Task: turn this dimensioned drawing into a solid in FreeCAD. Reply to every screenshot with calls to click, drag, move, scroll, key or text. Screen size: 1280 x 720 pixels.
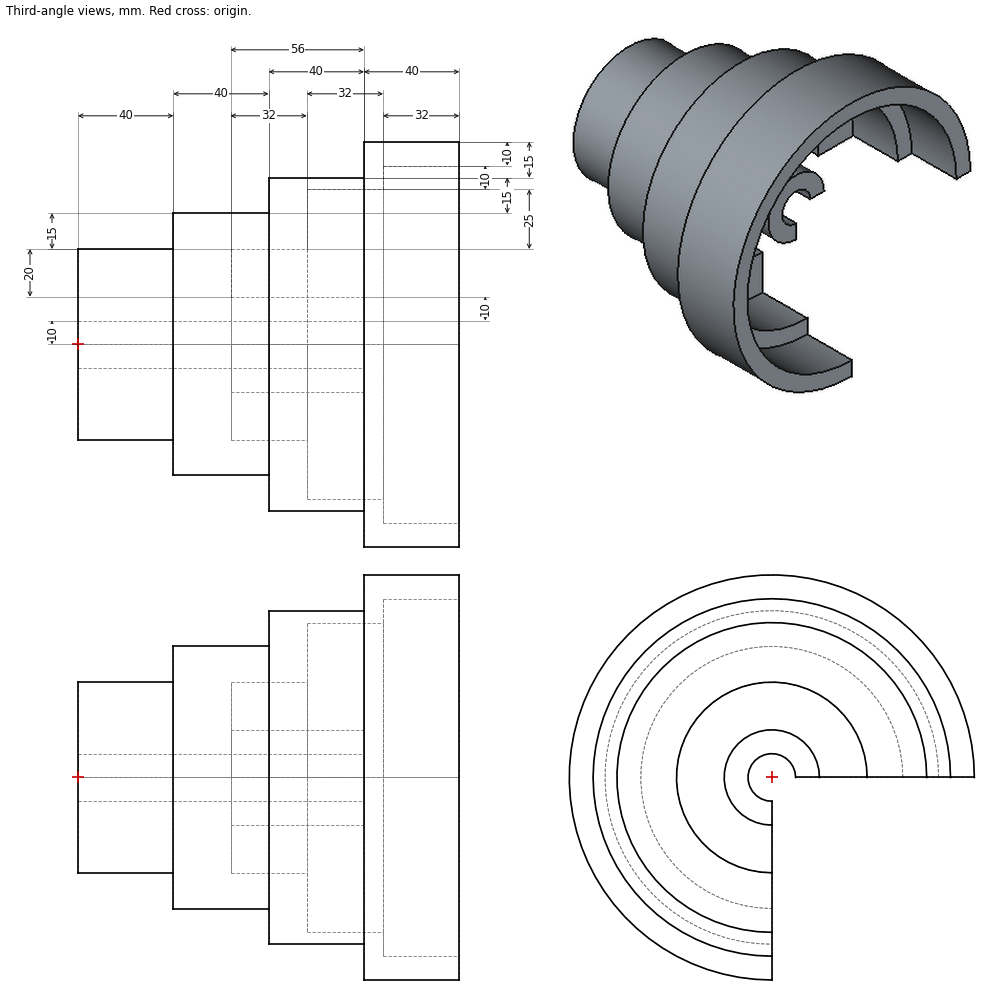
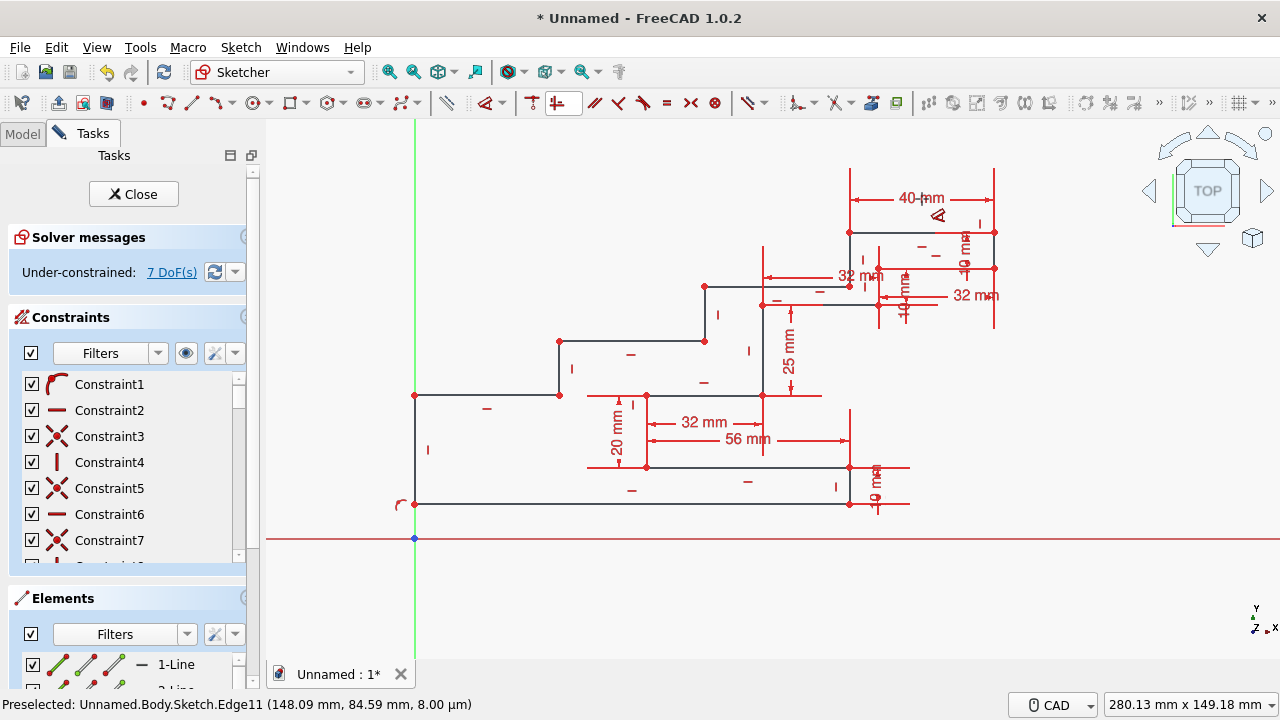
click(850, 249)
click(884, 247)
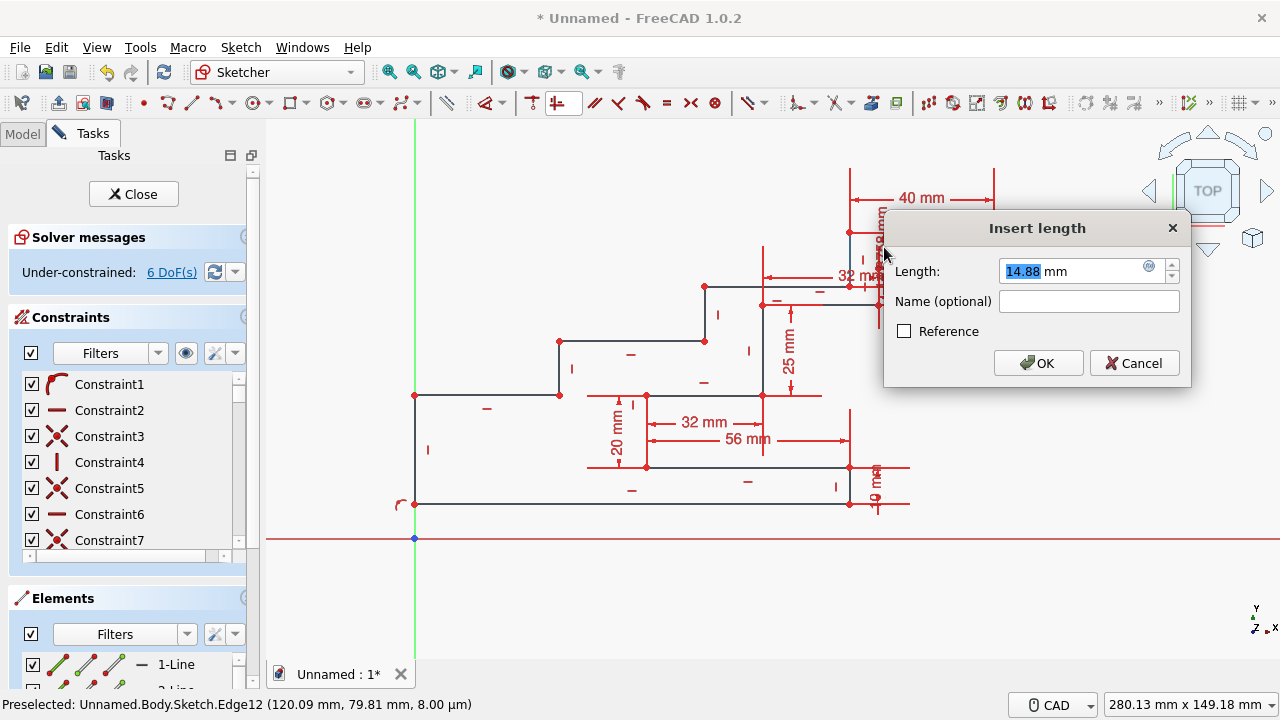
text(15)
key(Return)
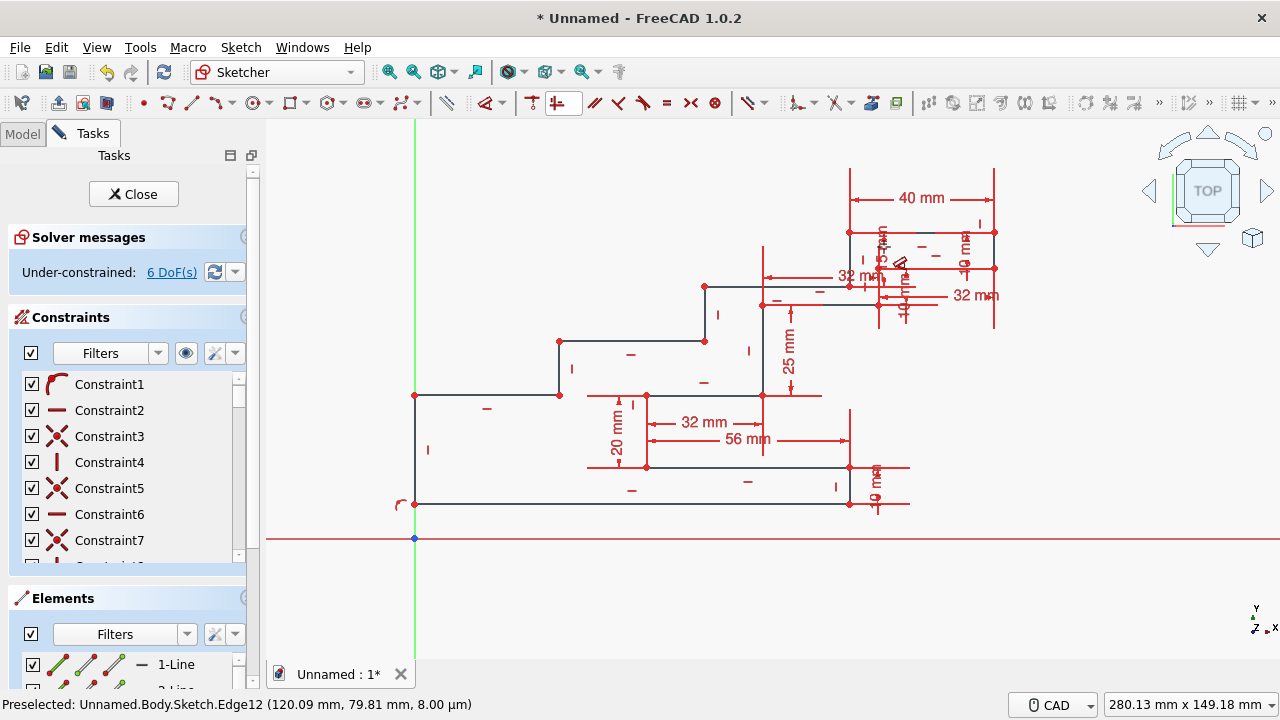
click(806, 287)
click(777, 253)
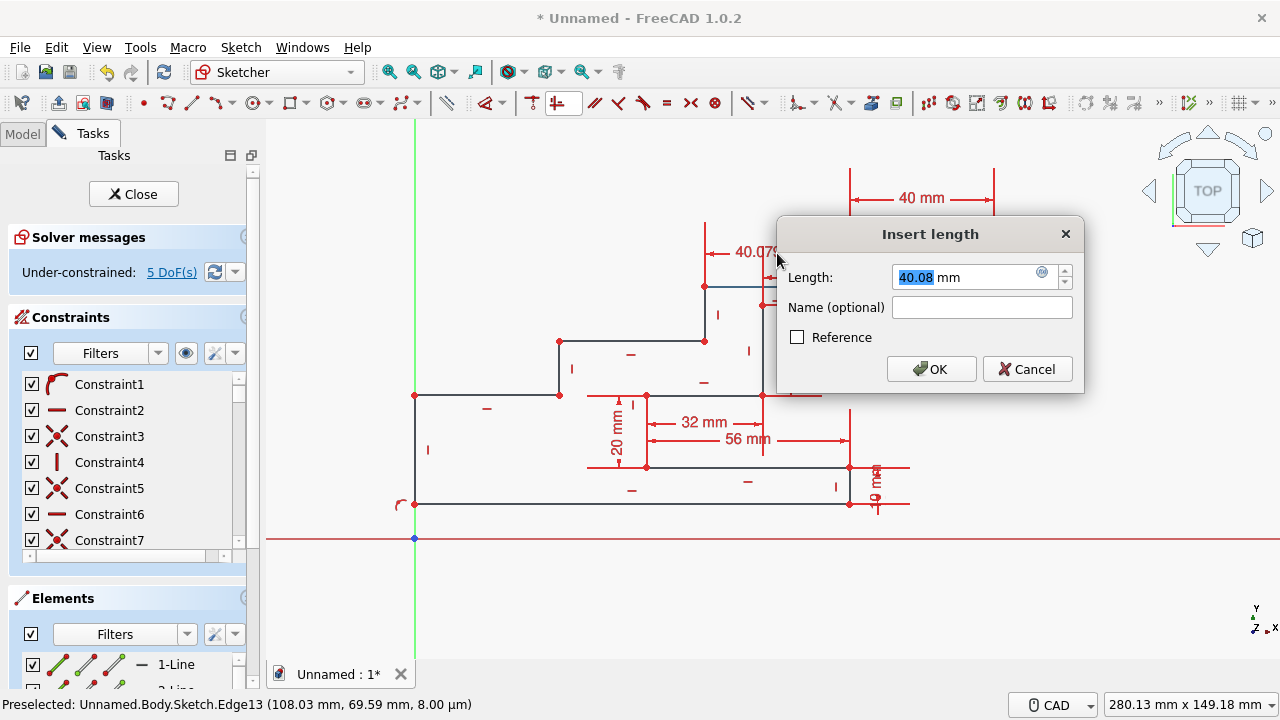
text(40)
key(Return)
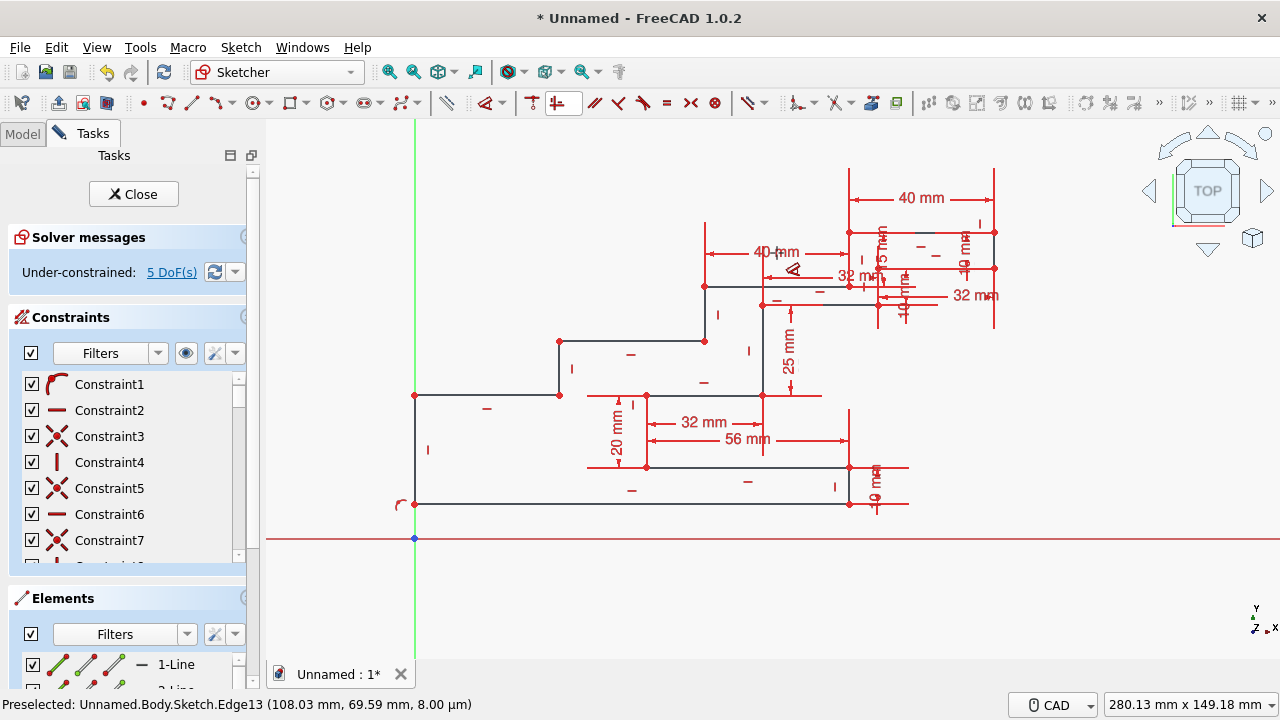
click(705, 303)
click(739, 314)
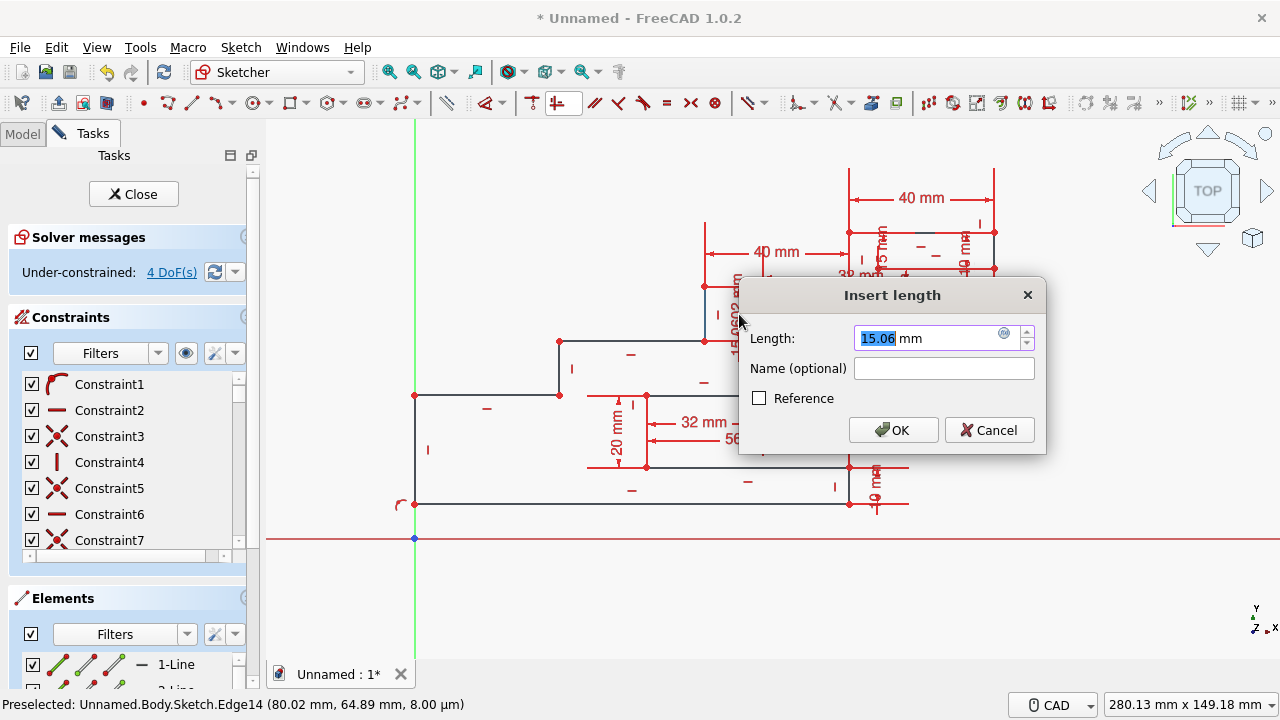
text(15)
key(Return)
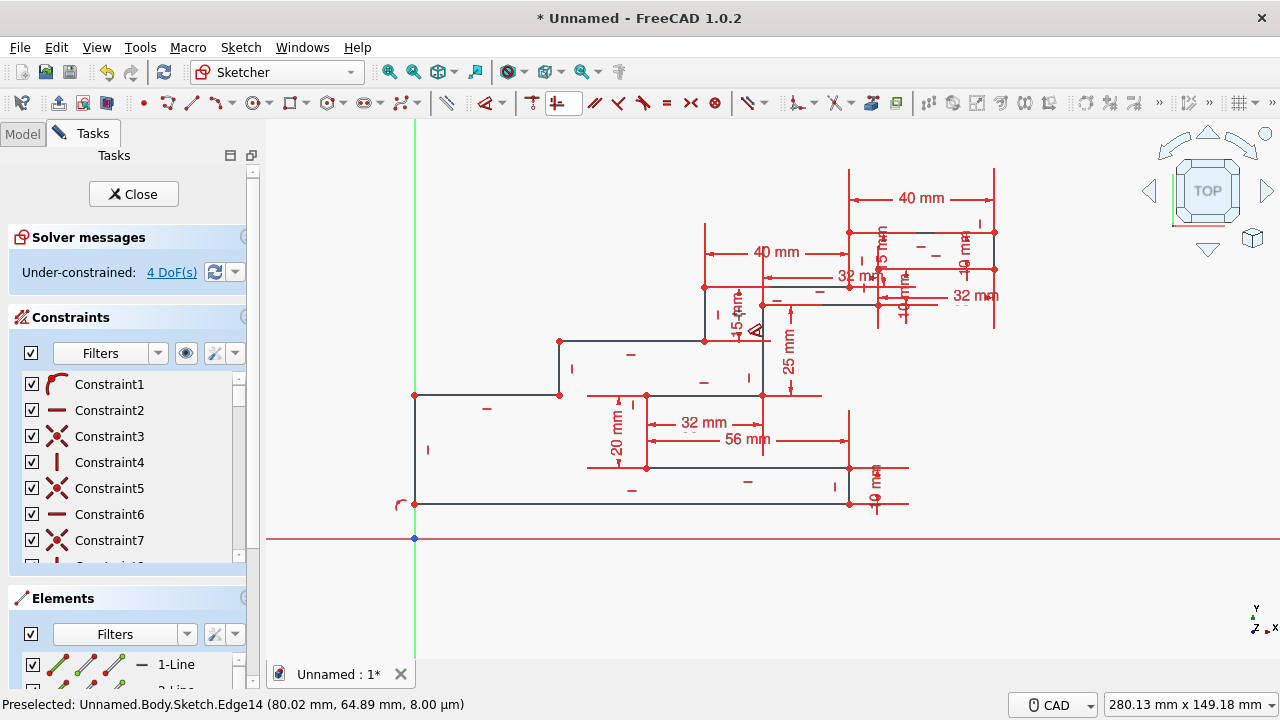
click(661, 341)
click(632, 307)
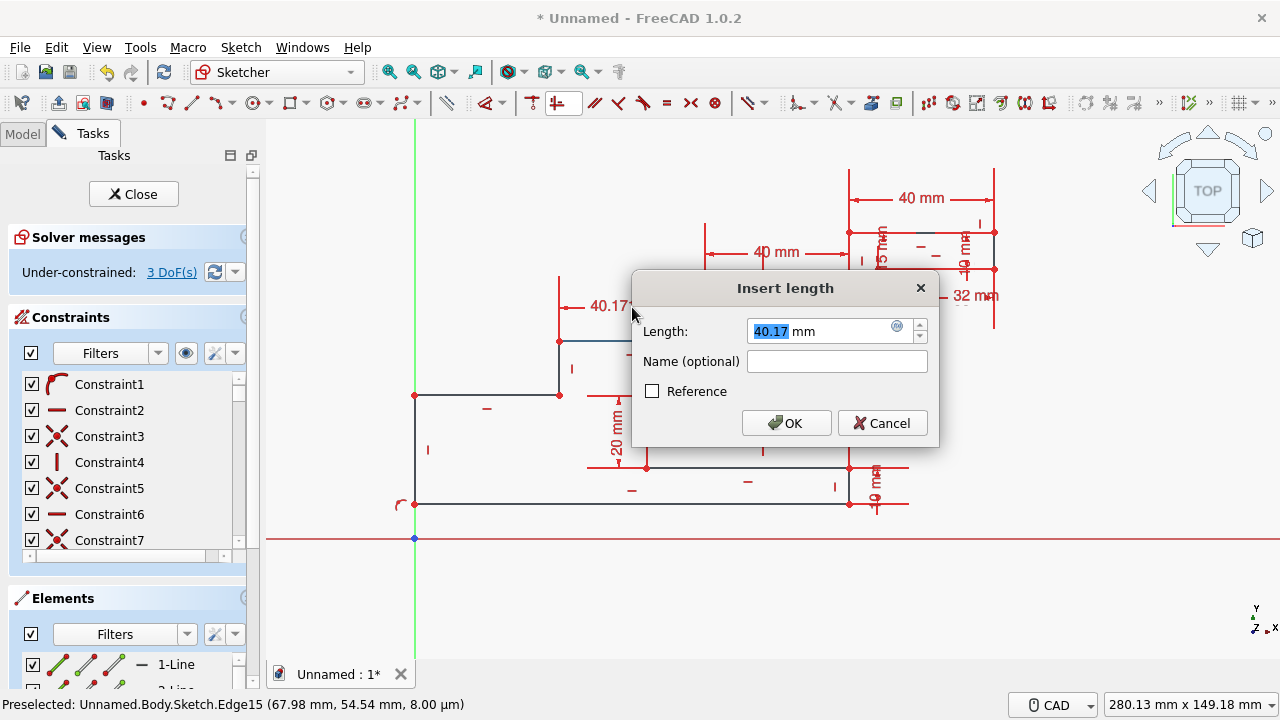
text(40)
key(Return)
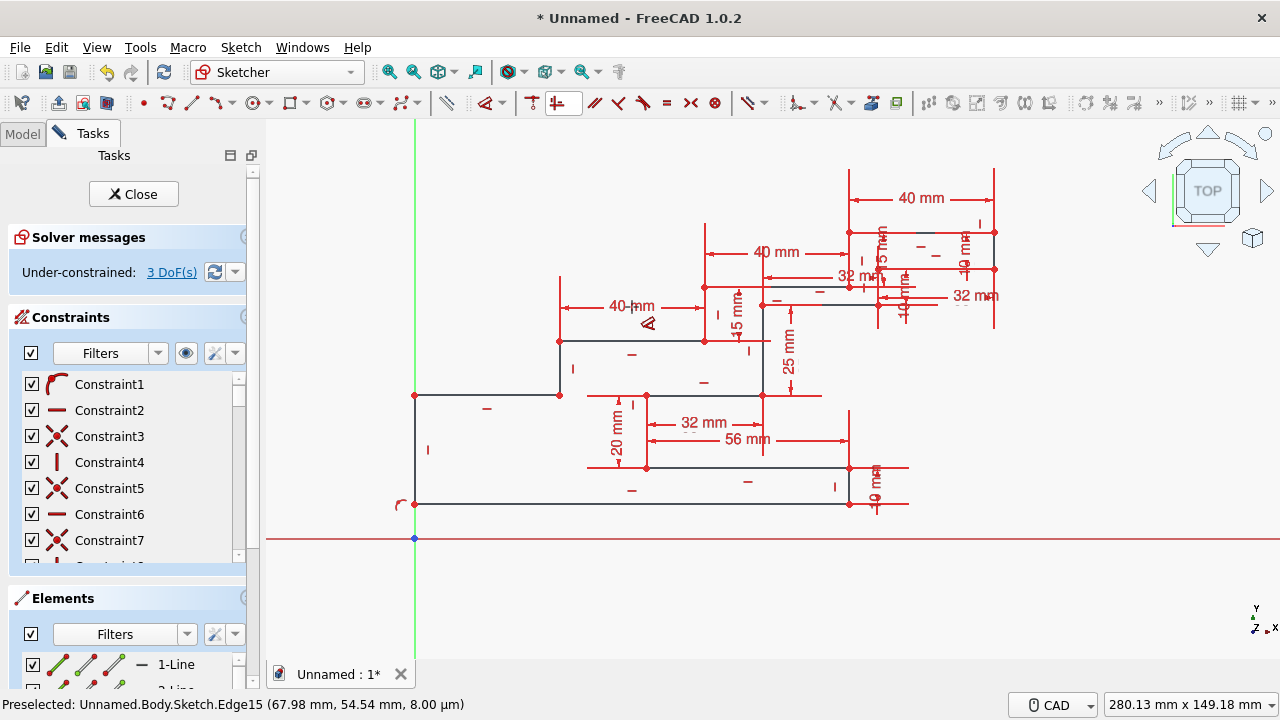
click(560, 358)
click(526, 368)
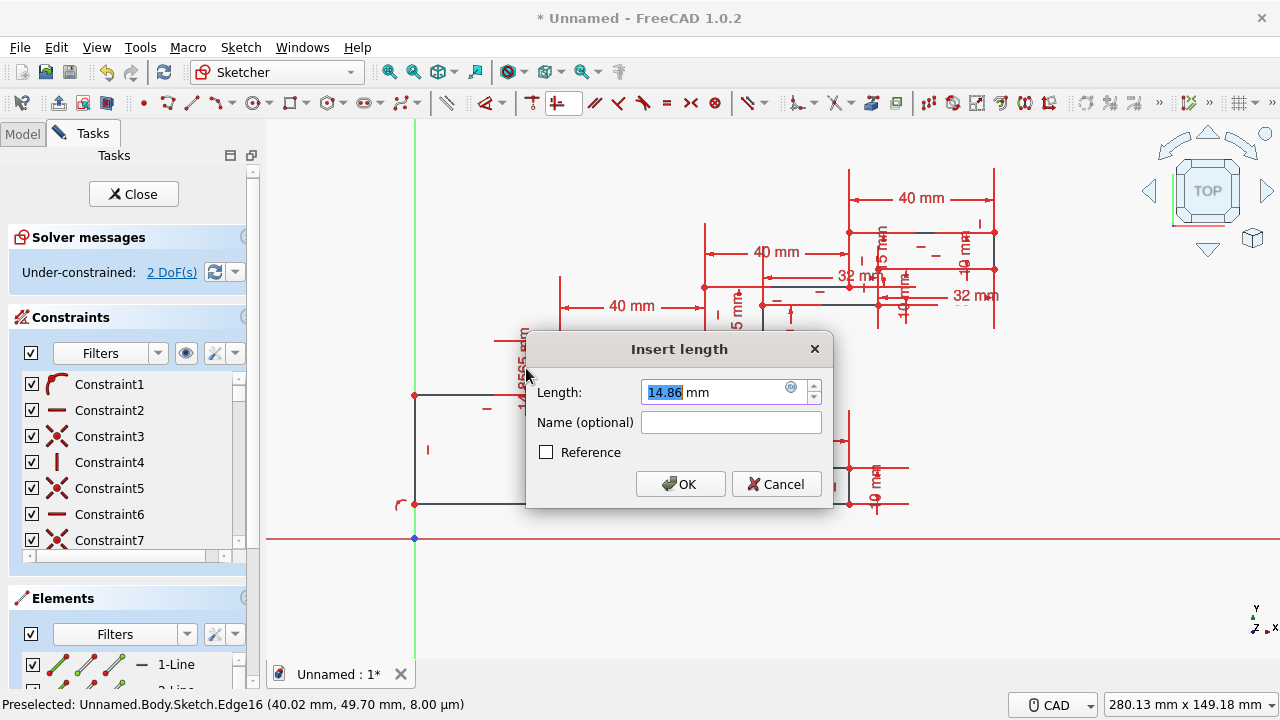
text(15)
key(Return)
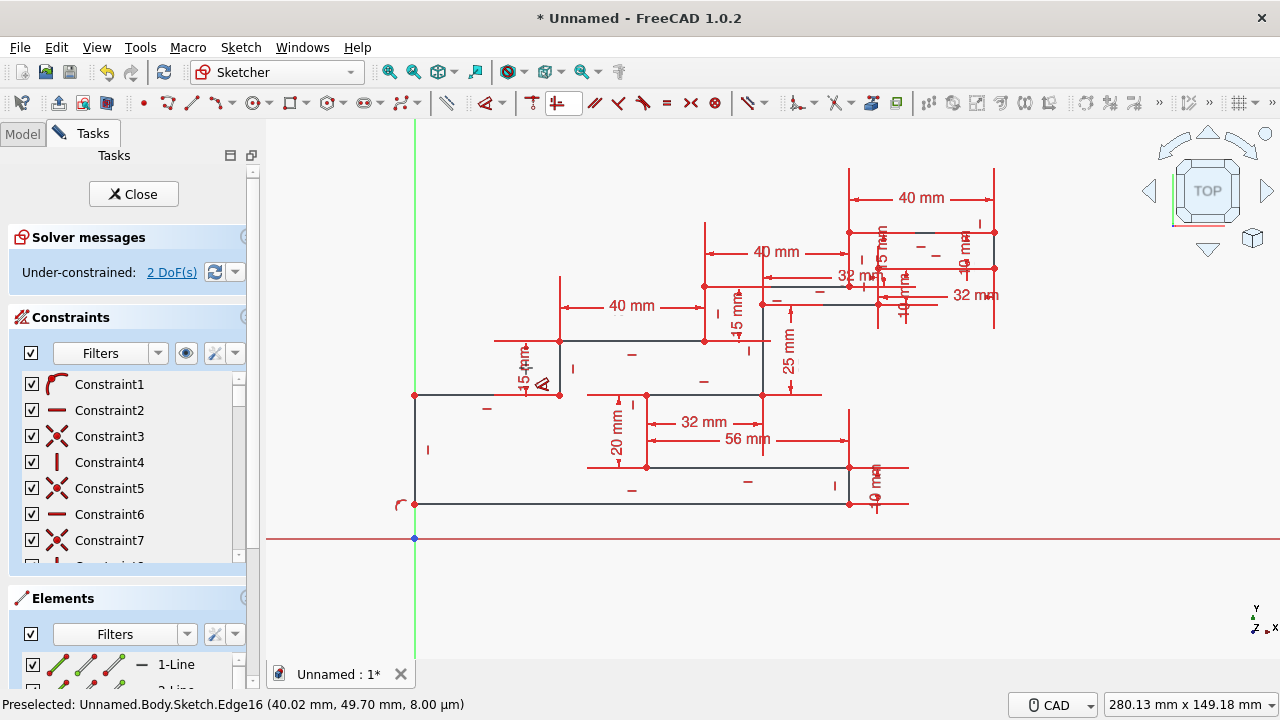
click(516, 395)
click(487, 429)